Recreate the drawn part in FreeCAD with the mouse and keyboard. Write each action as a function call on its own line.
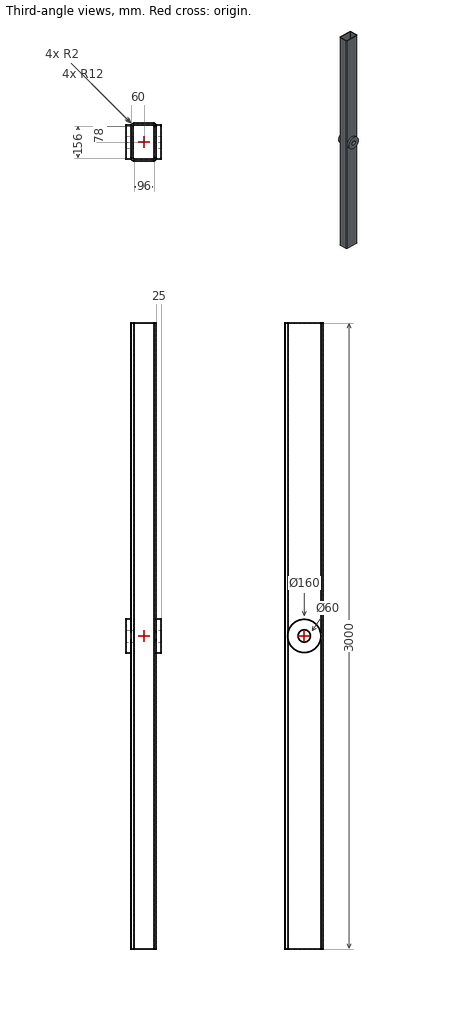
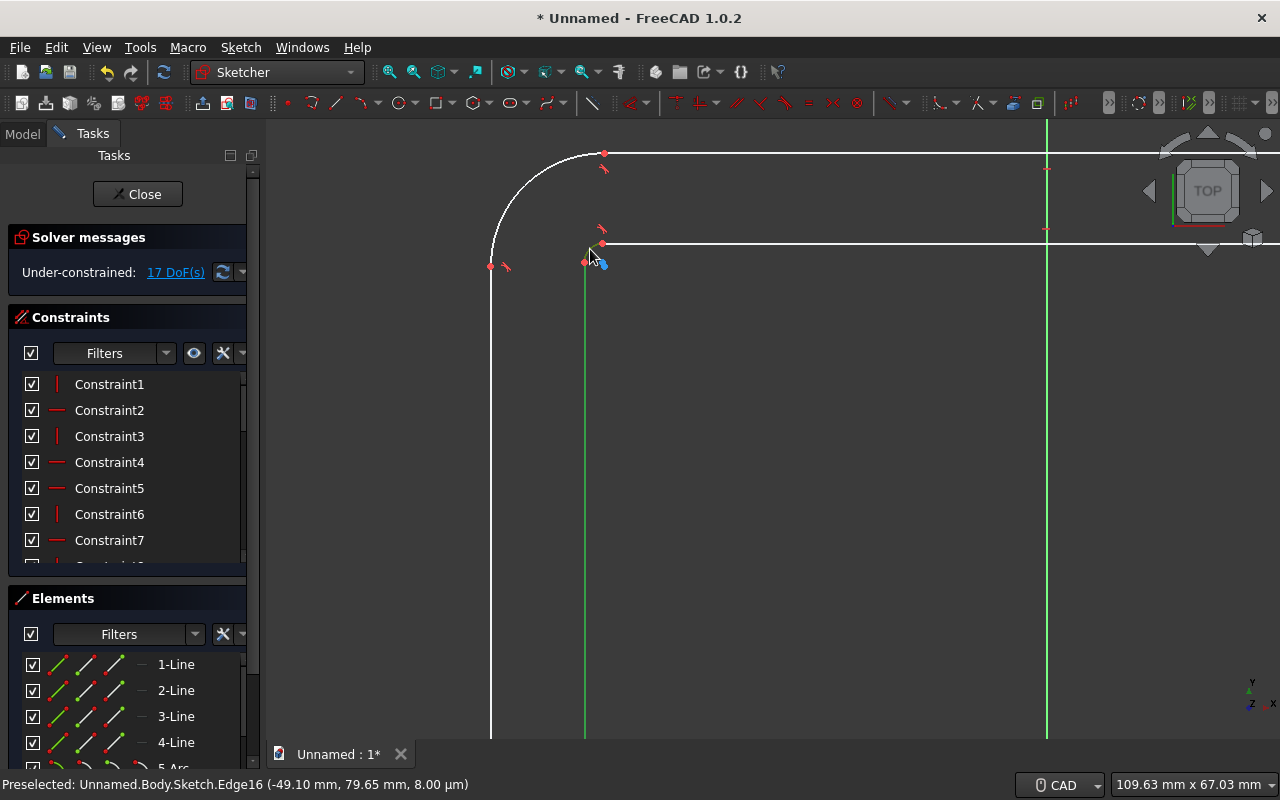
click(786, 104)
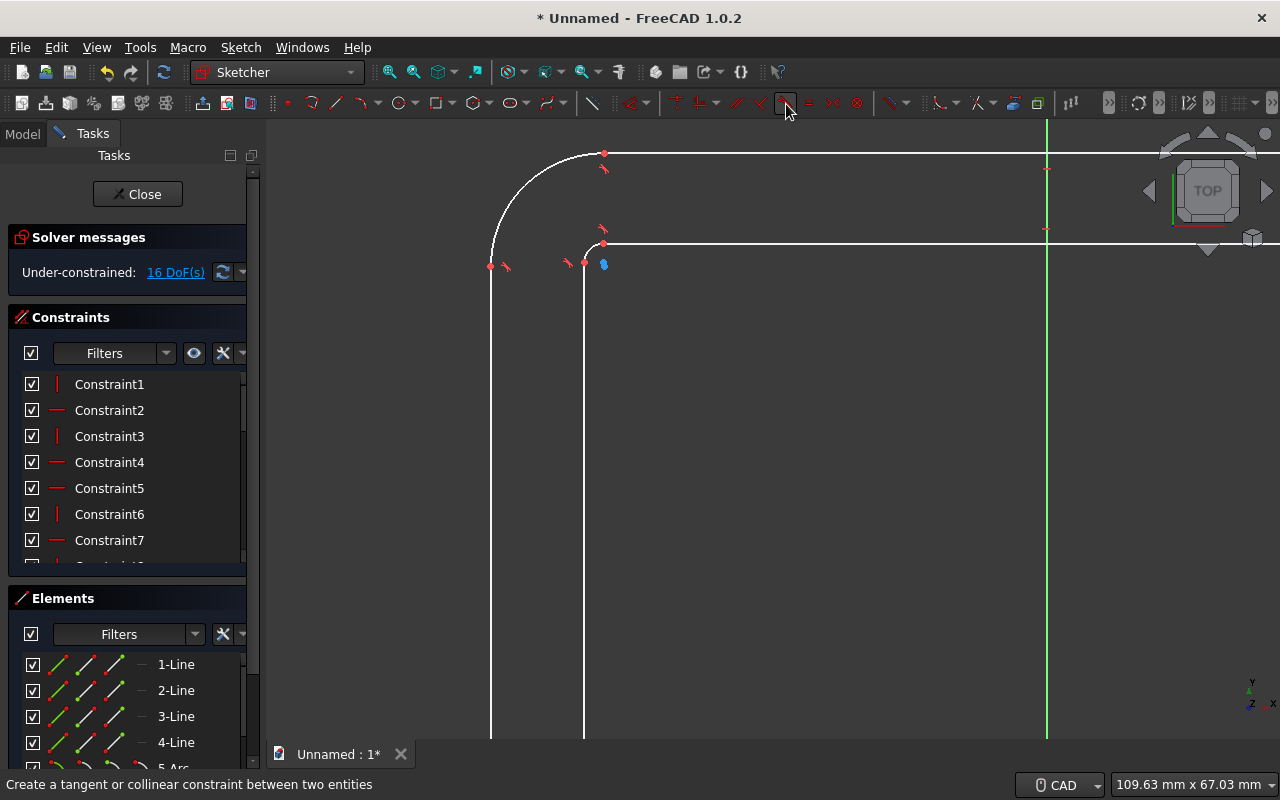
scroll(592, 248, down, 7)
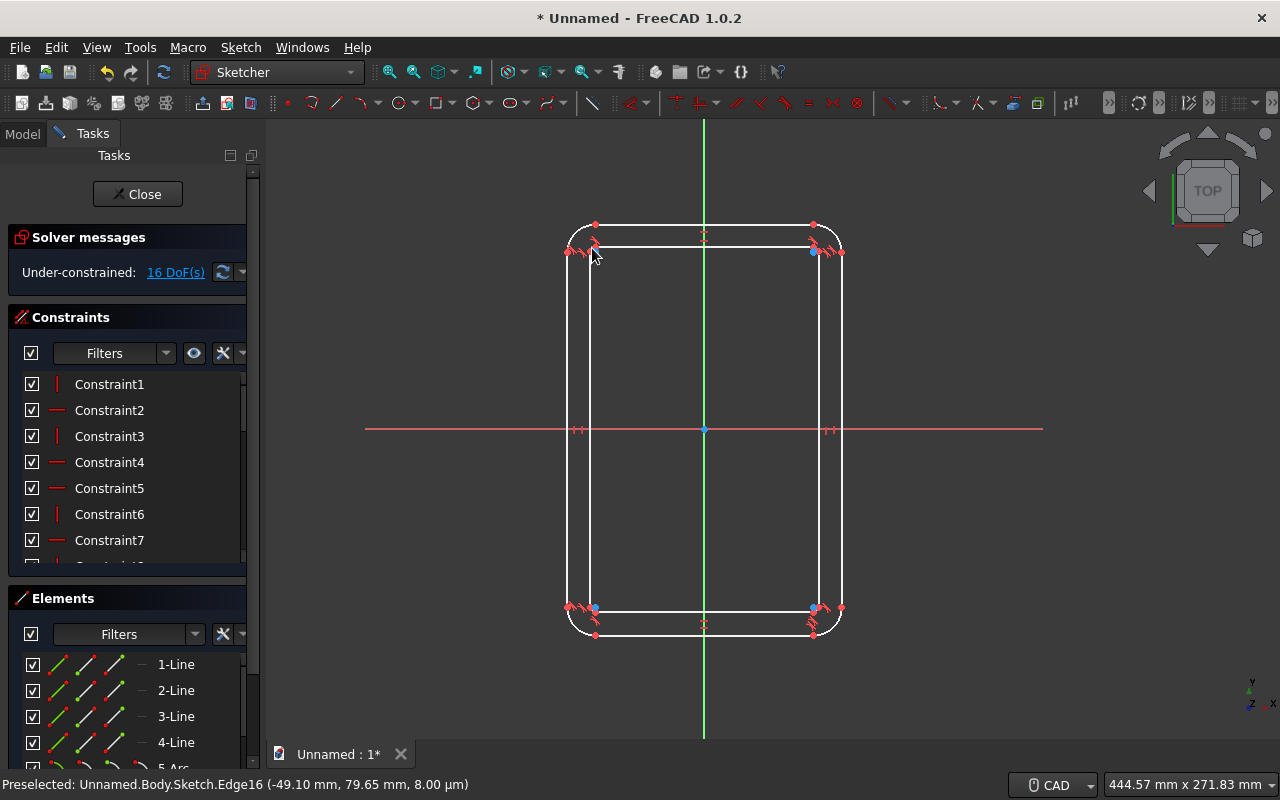
click(839, 240)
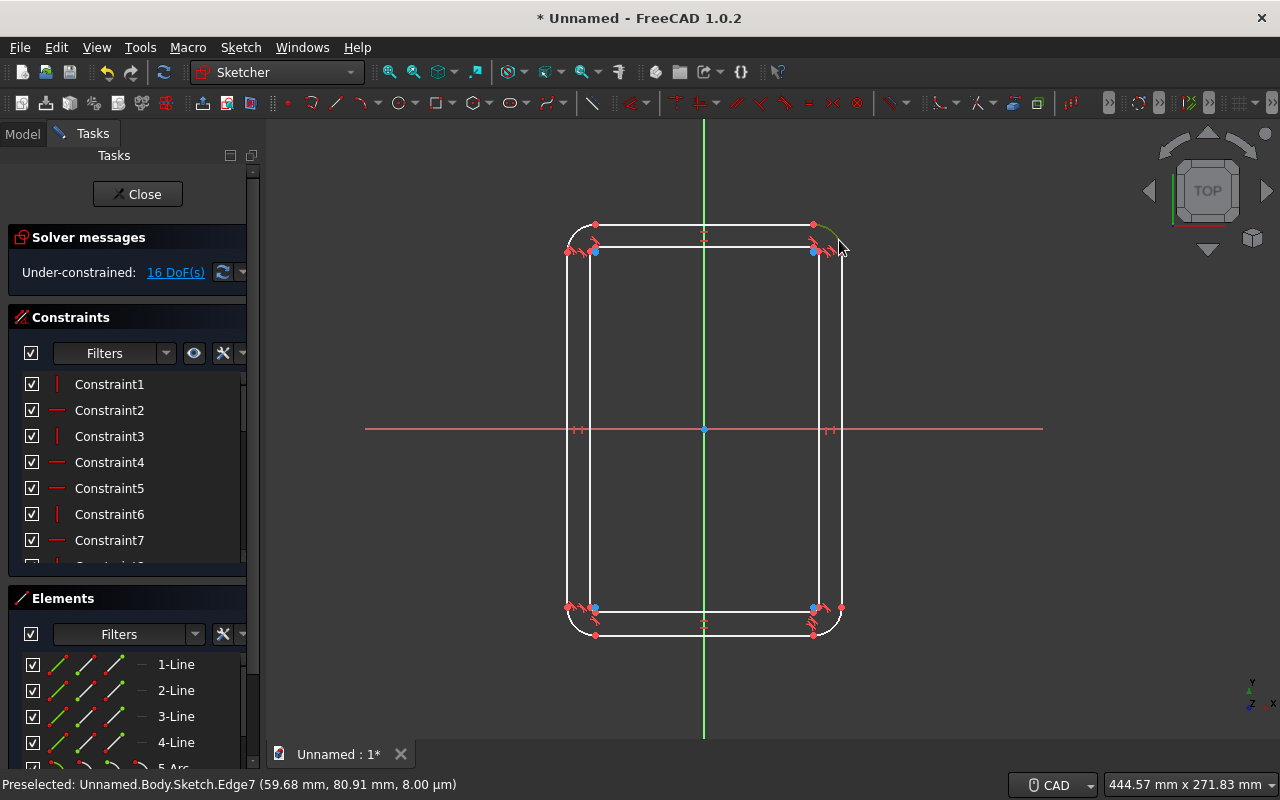
scroll(817, 248, up, 7)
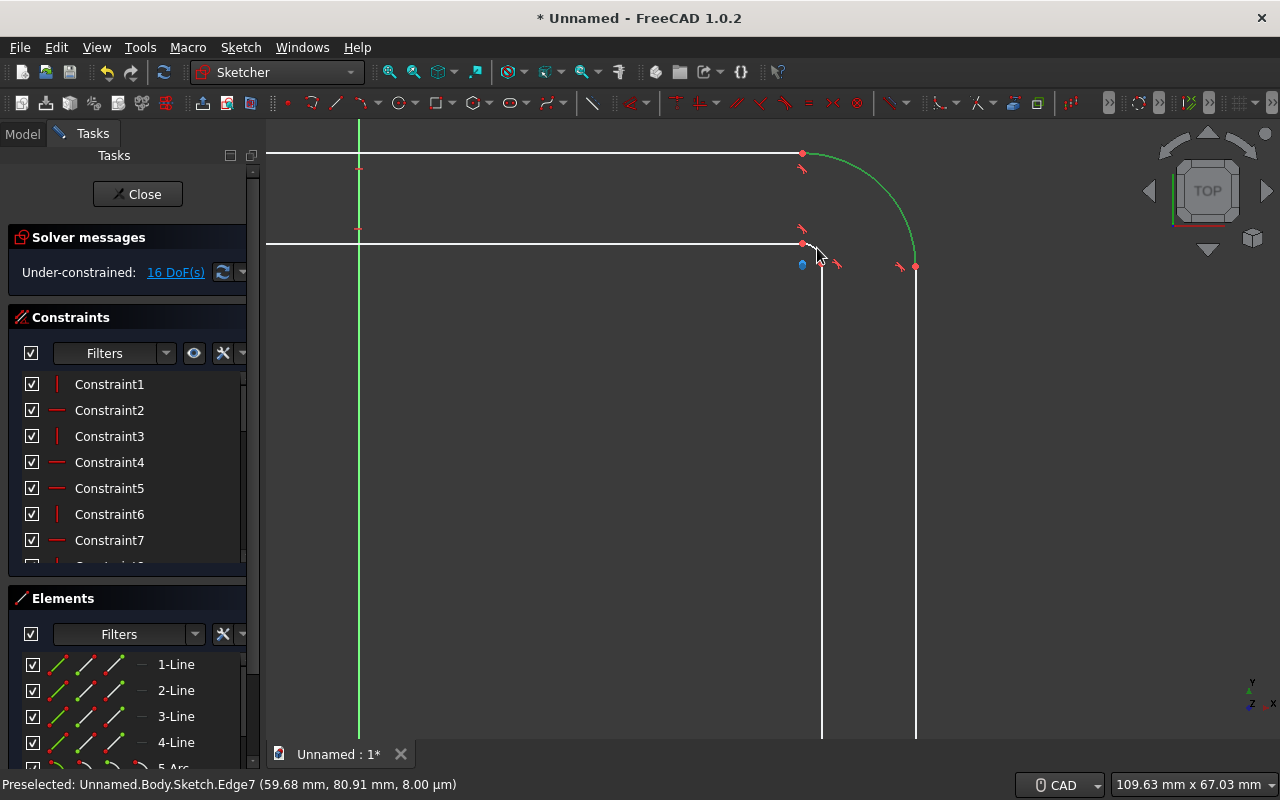
click(816, 249)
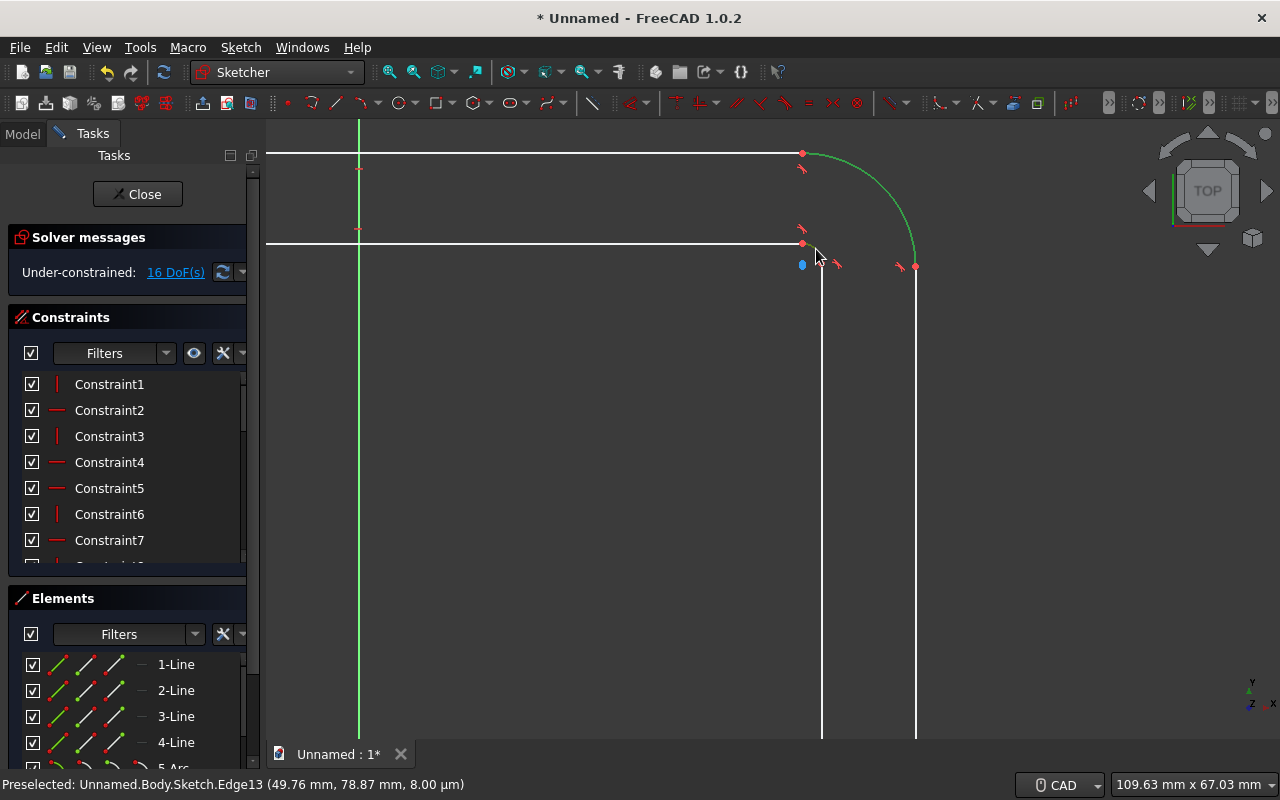
click(676, 104)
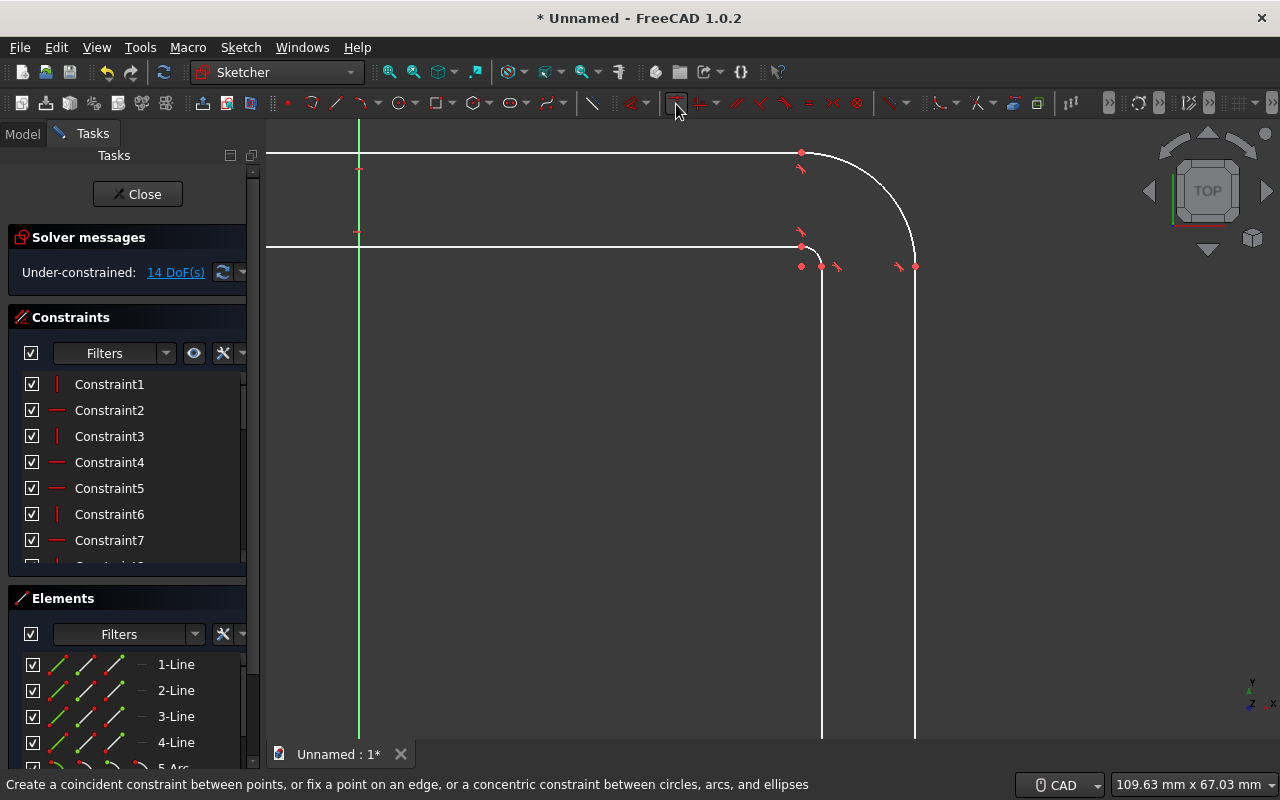
scroll(818, 248, down, 7)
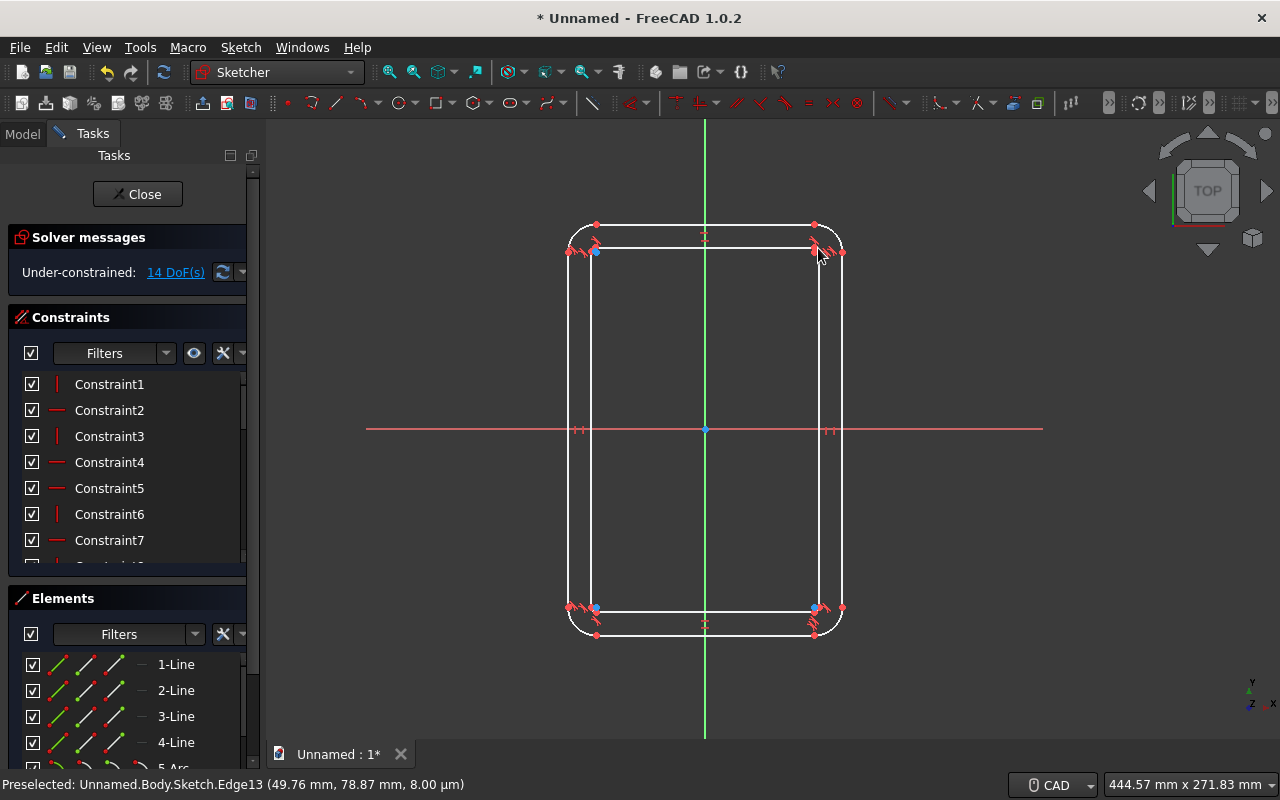
click(827, 632)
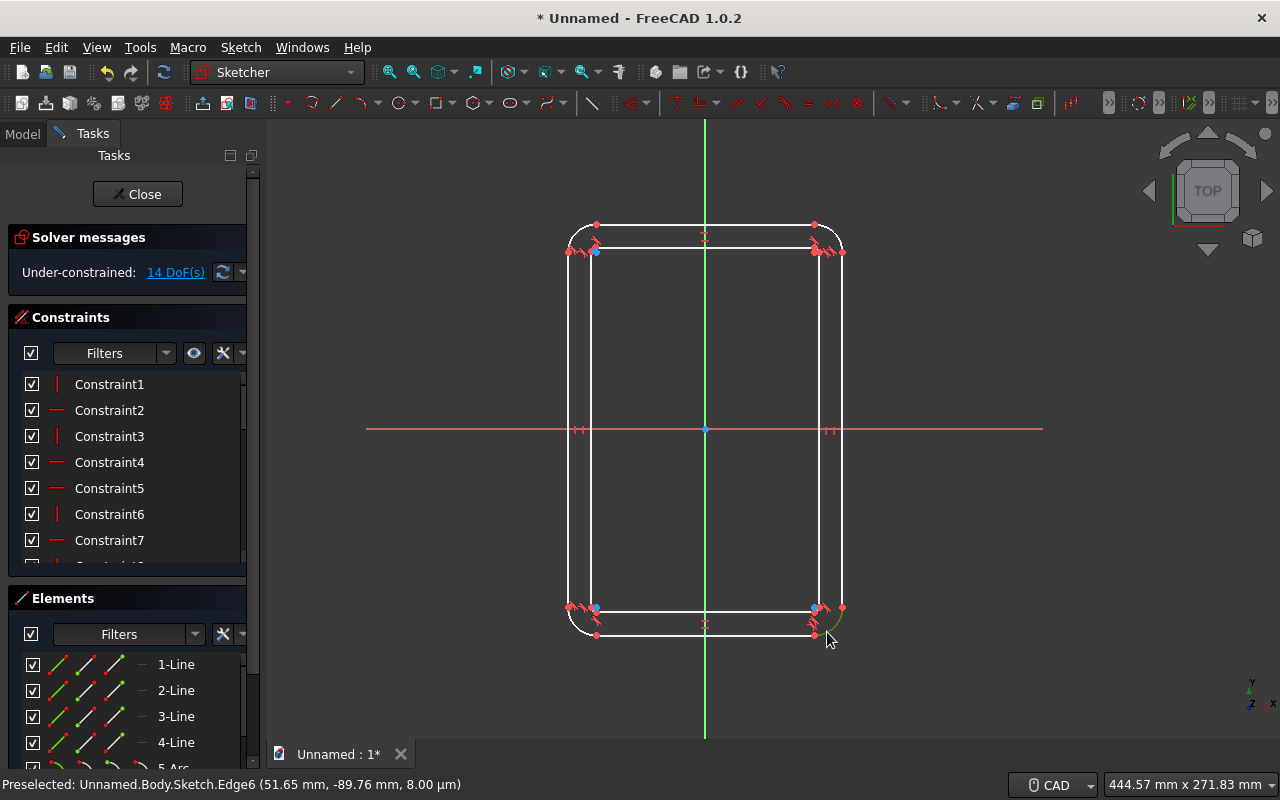
scroll(818, 611, up, 7)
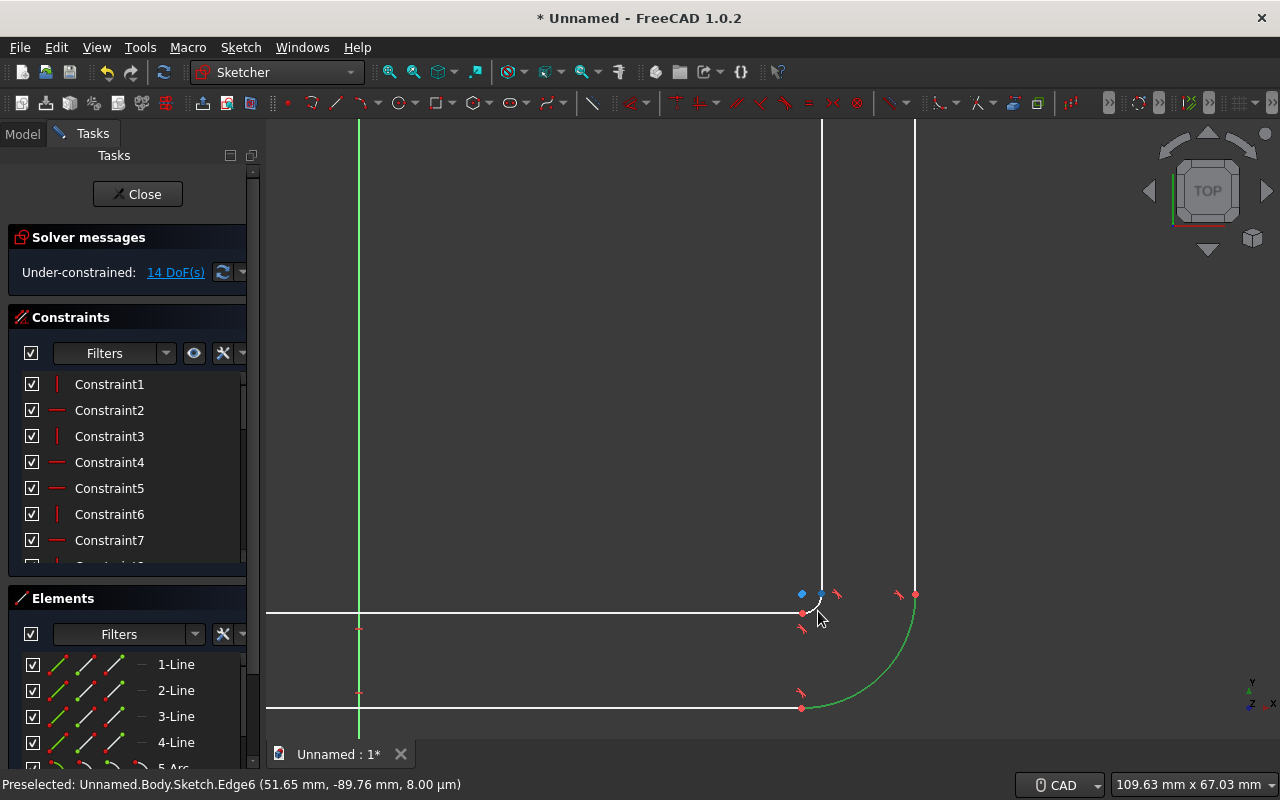
click(816, 608)